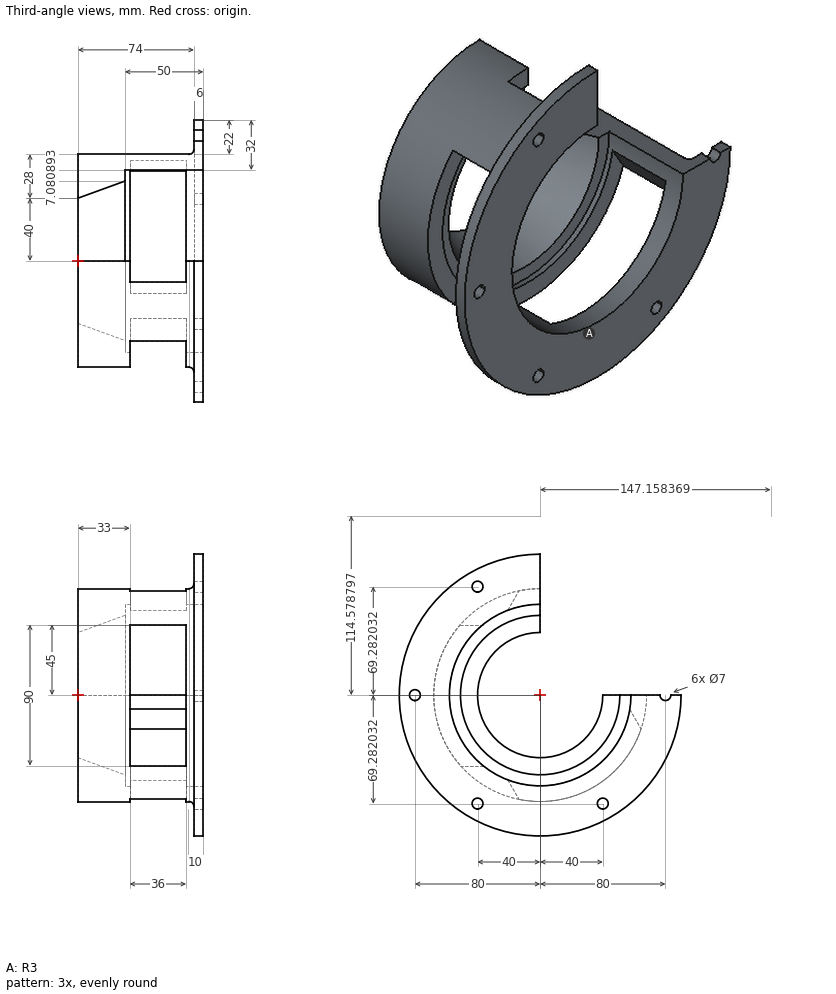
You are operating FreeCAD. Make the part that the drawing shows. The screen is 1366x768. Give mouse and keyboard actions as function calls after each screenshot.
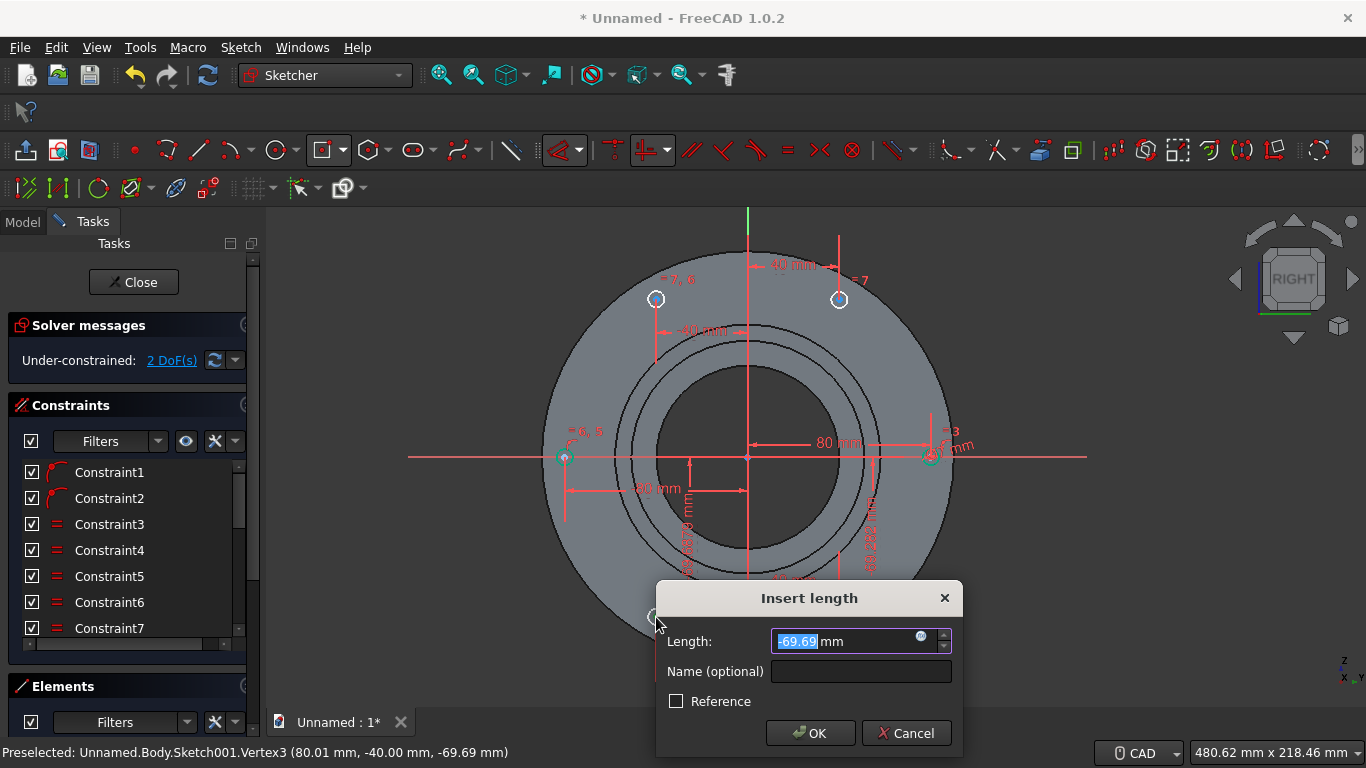
text(-69.282032)
key(Return)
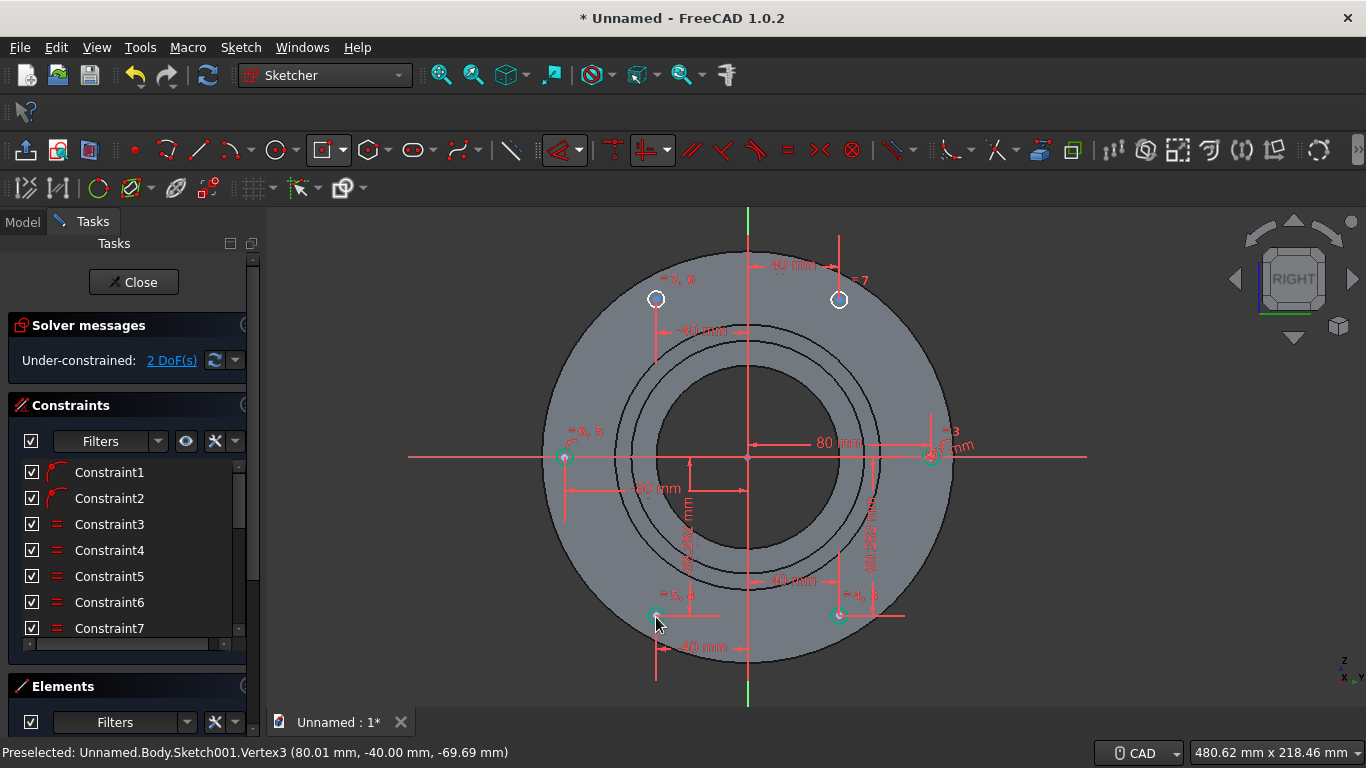
click(656, 299)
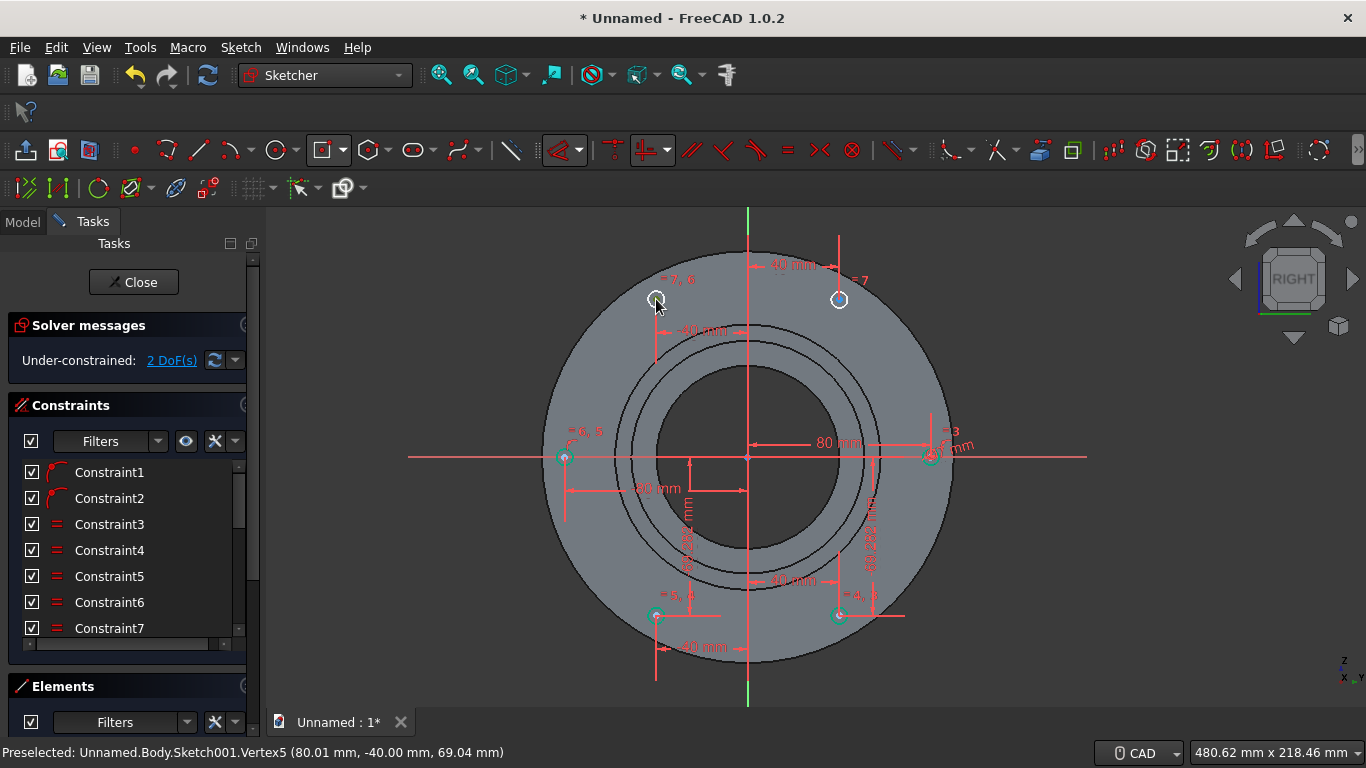
key(i)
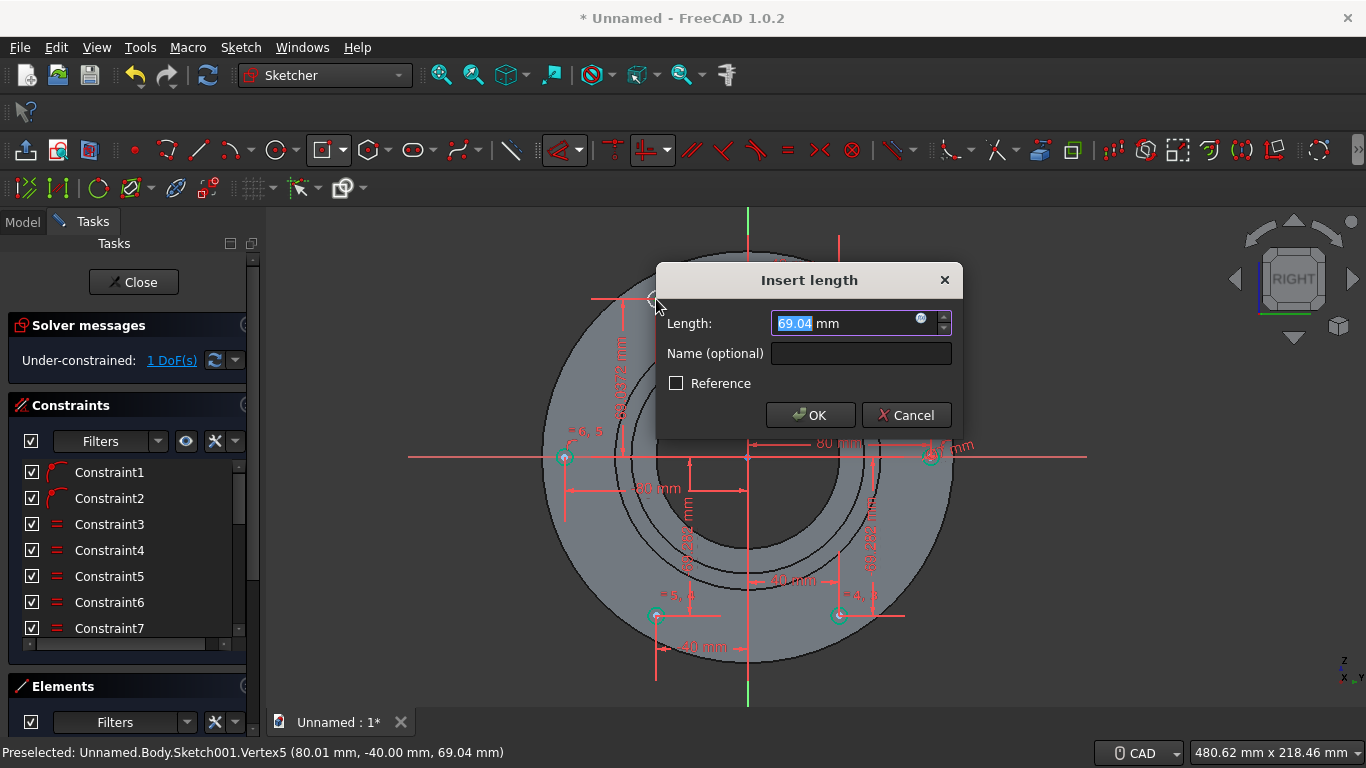
text(69.282032)
key(Return)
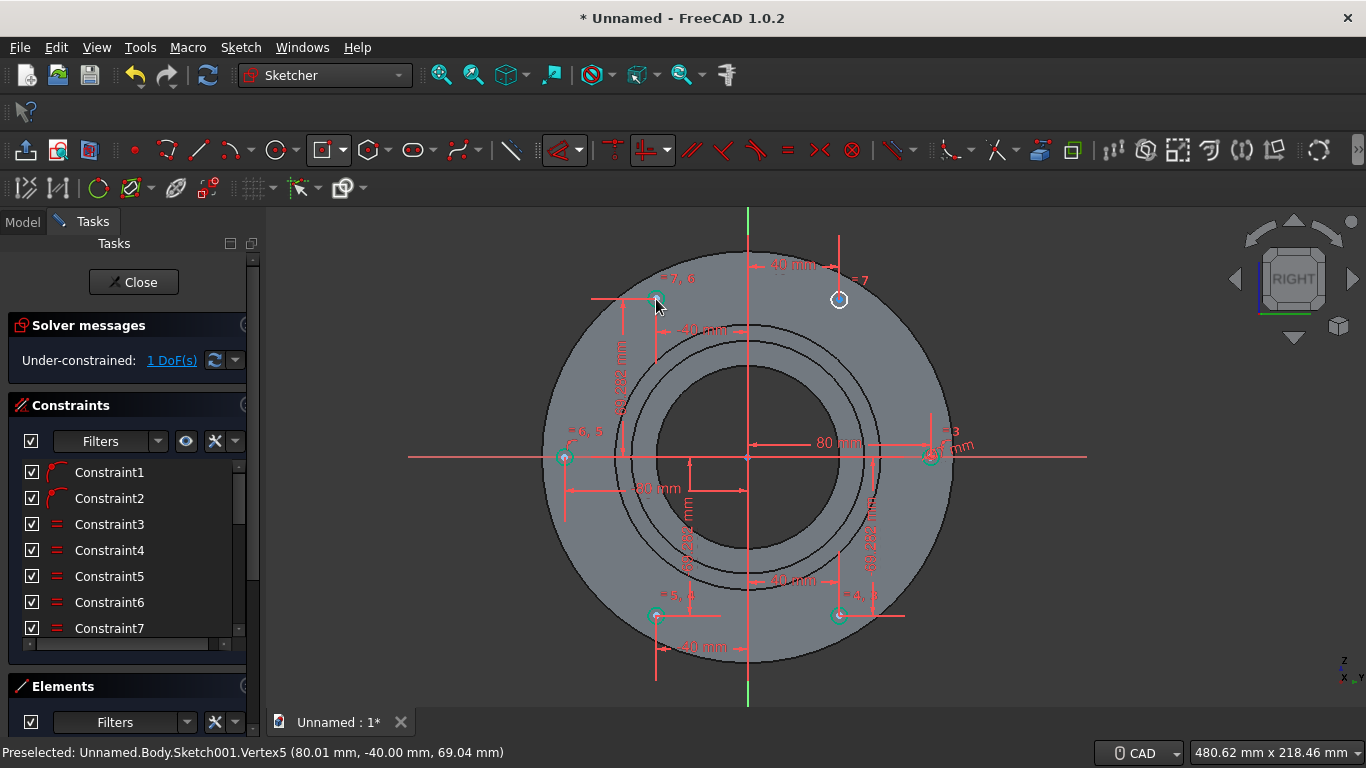
click(839, 300)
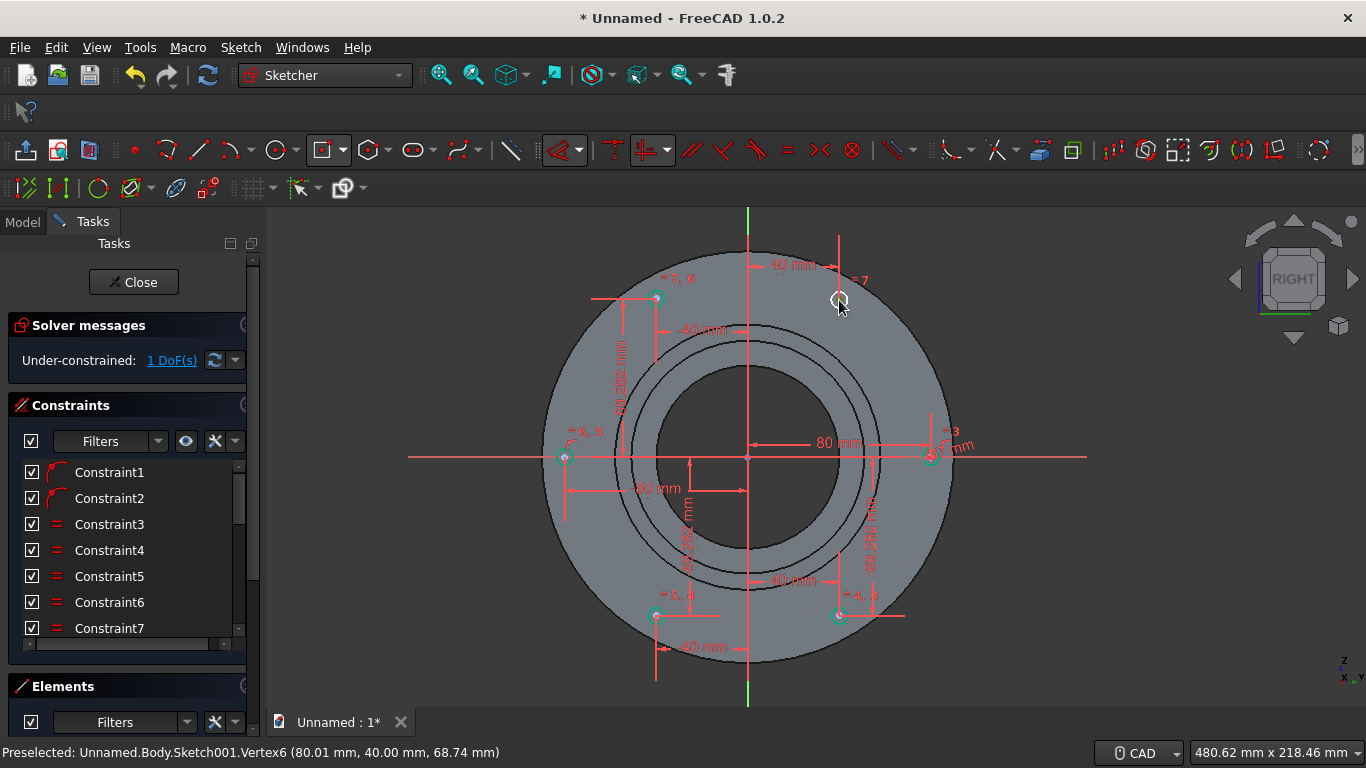
key(i)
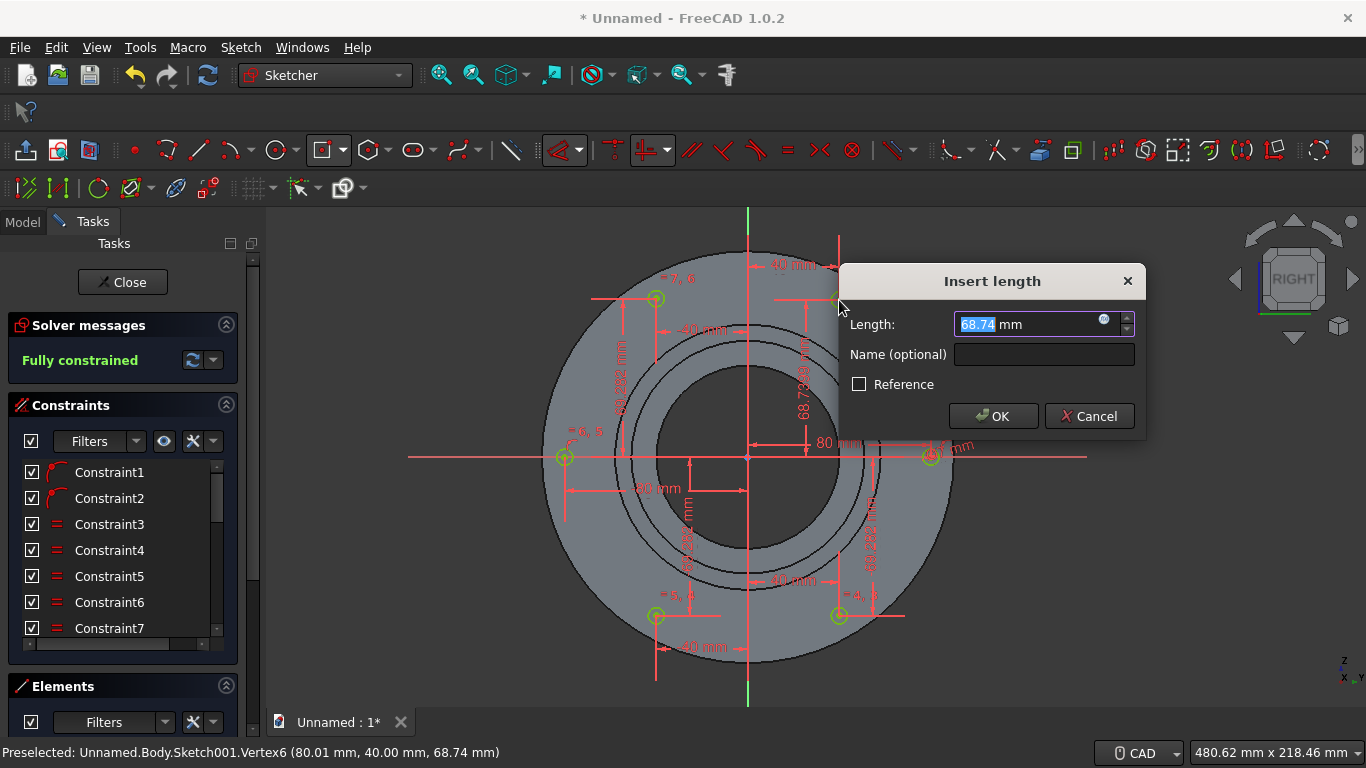
text(69.282032)
key(Return)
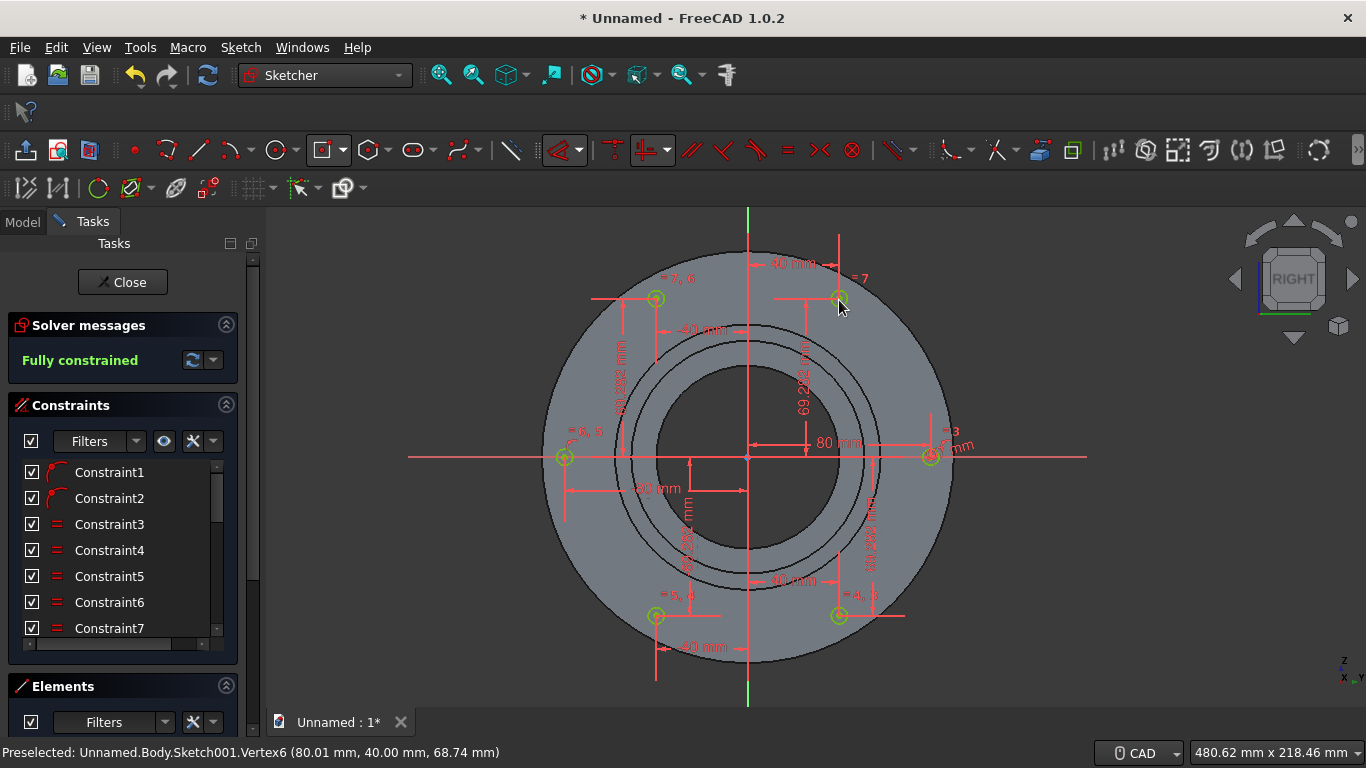
click(123, 282)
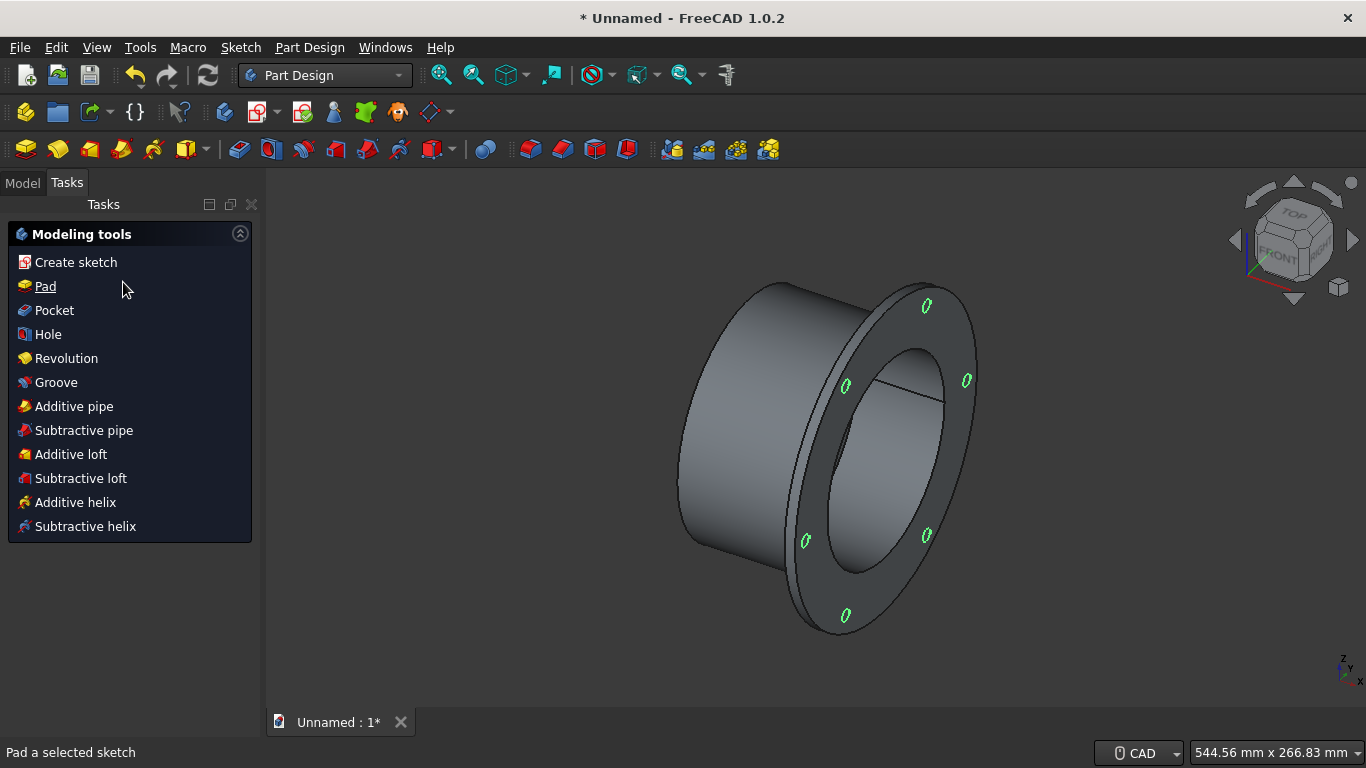
click(240, 150)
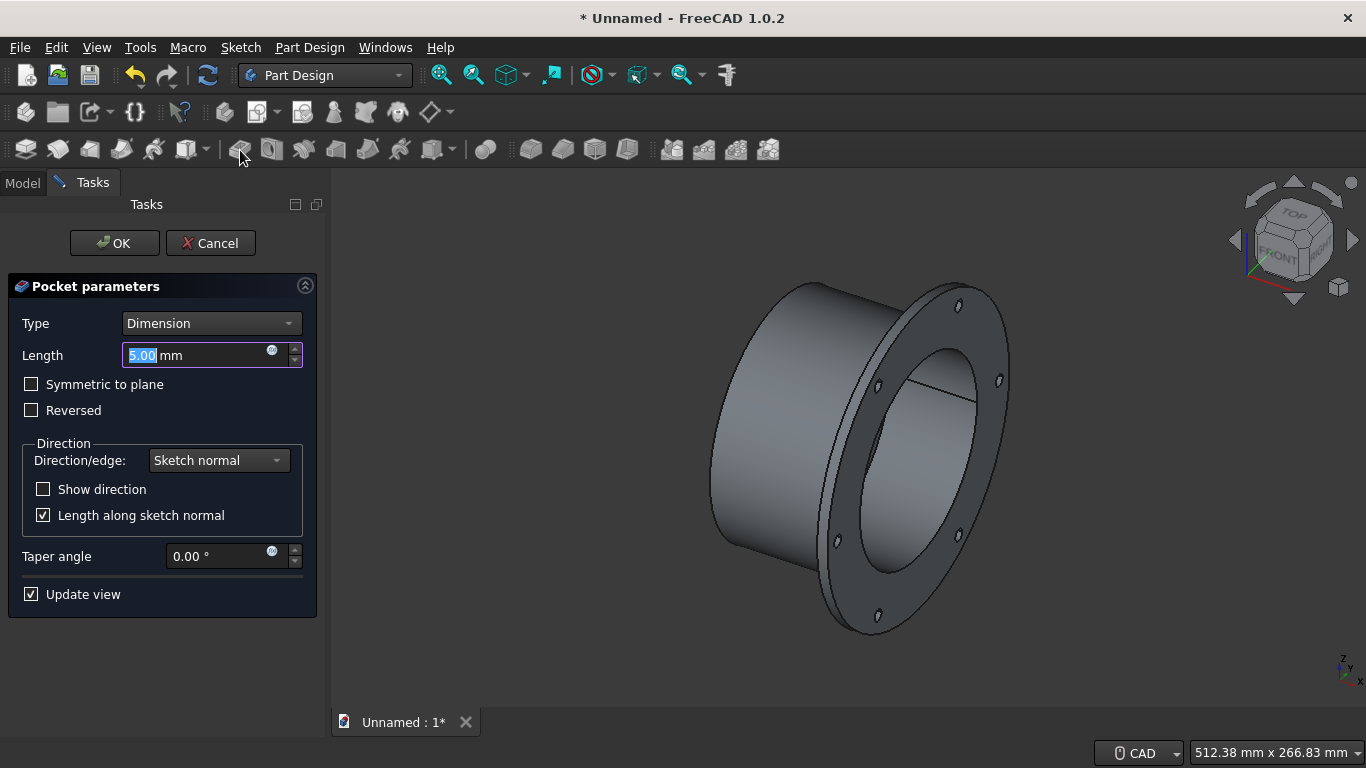
text(10)
key(Tab)